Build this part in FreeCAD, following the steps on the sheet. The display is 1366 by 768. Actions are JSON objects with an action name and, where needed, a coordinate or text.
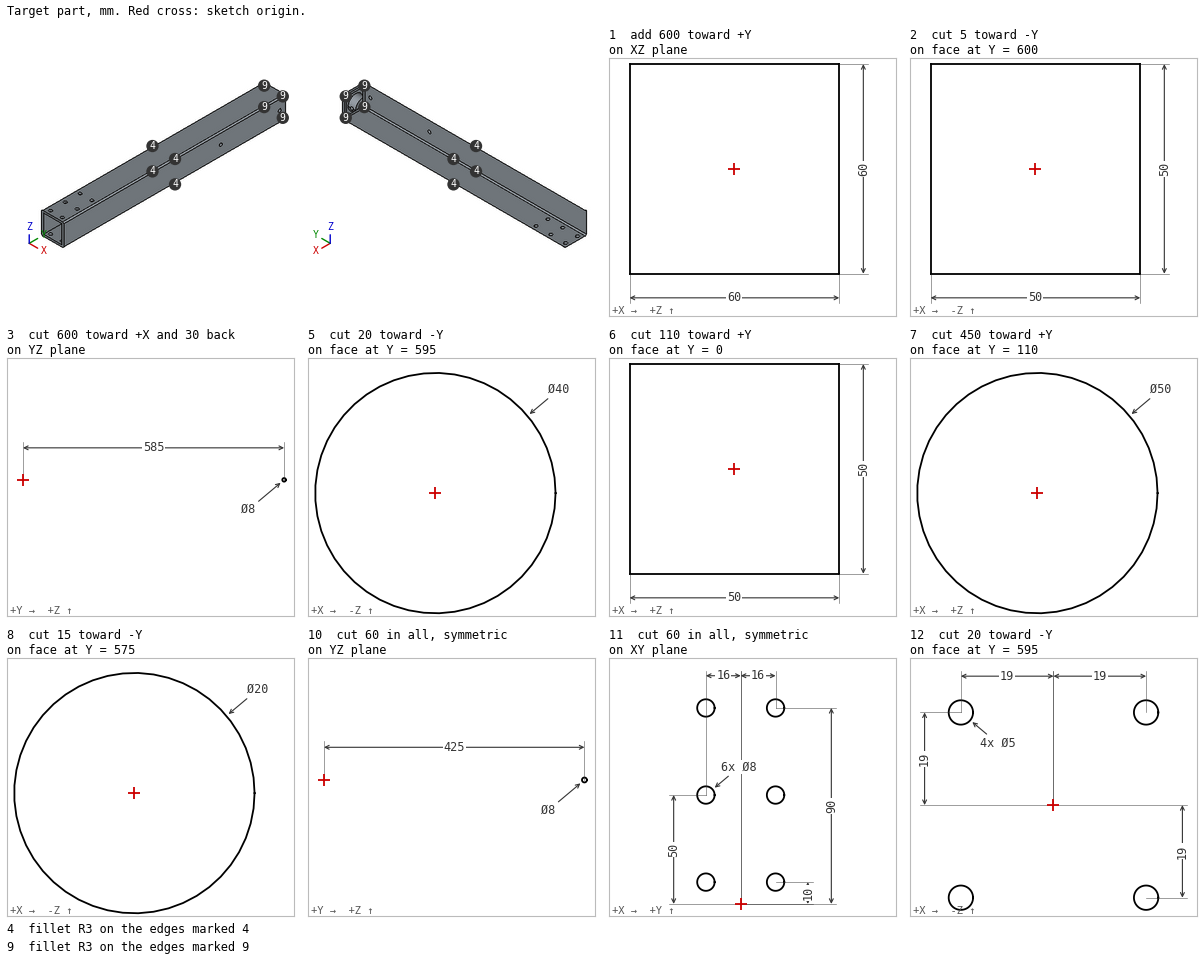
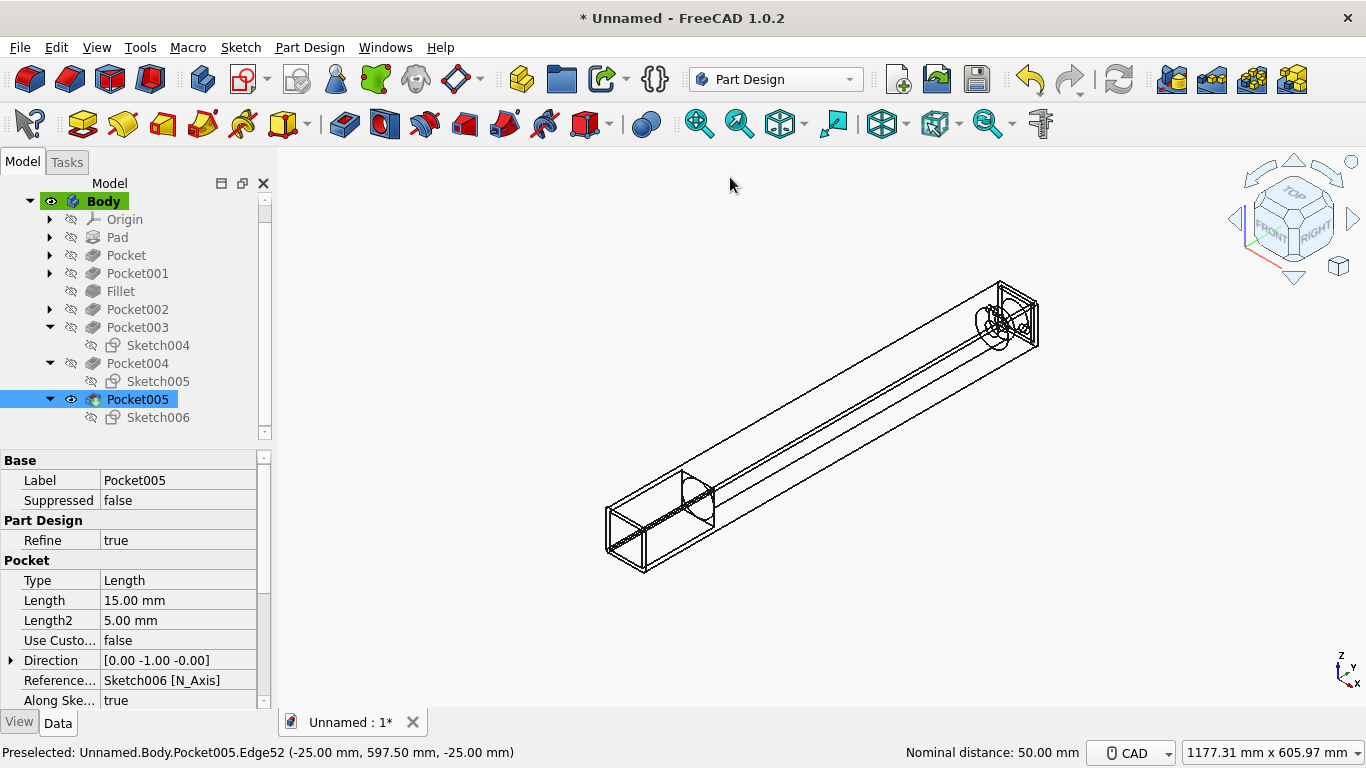
{"action": "key", "text": "2"}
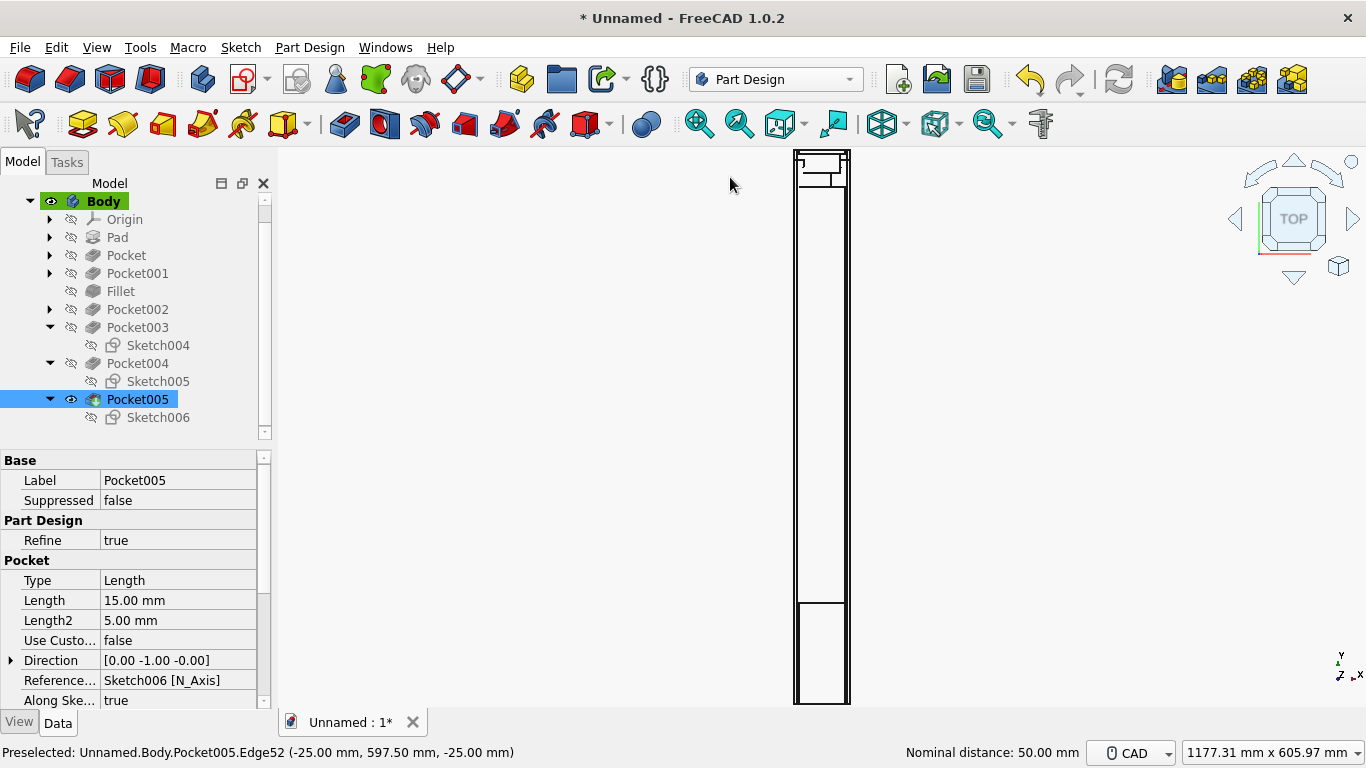
{"action": "key", "text": "1"}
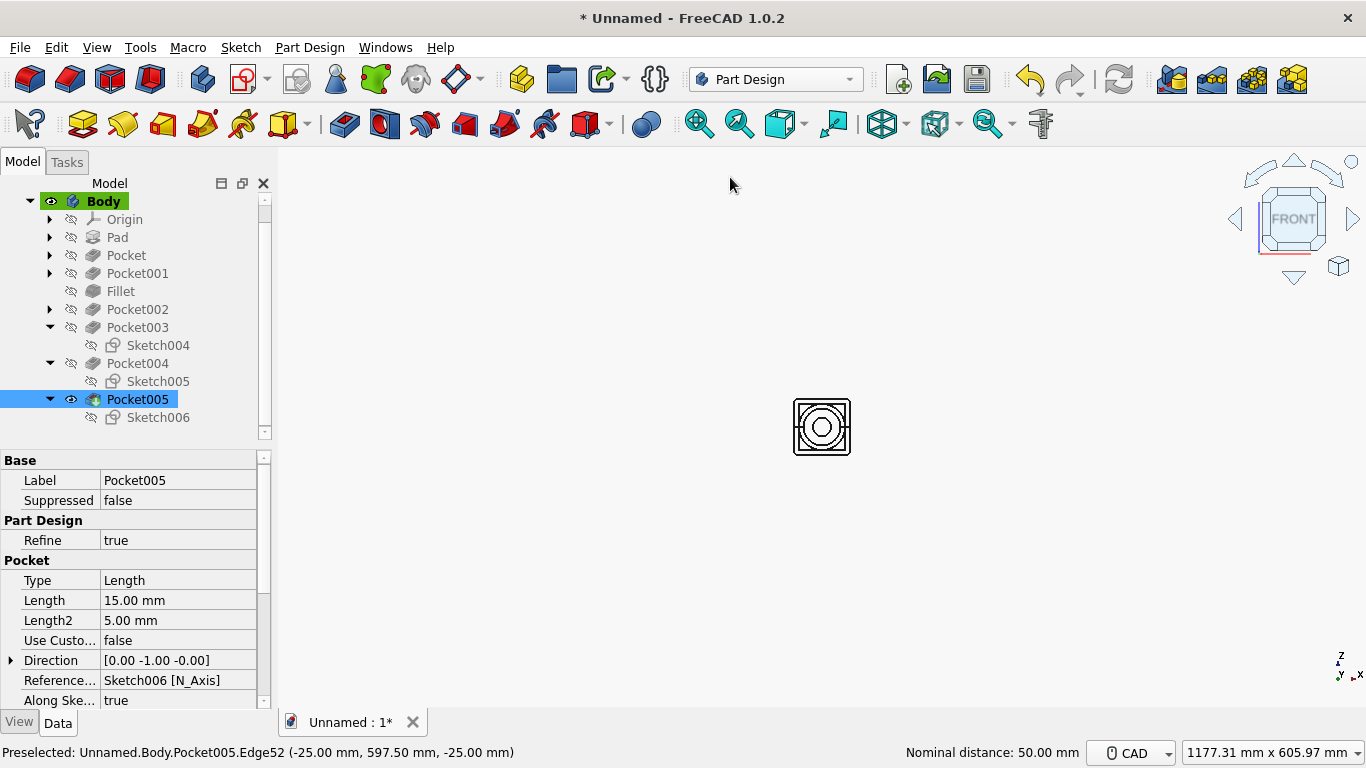
{"action": "left_click", "coordinate": [700, 124]}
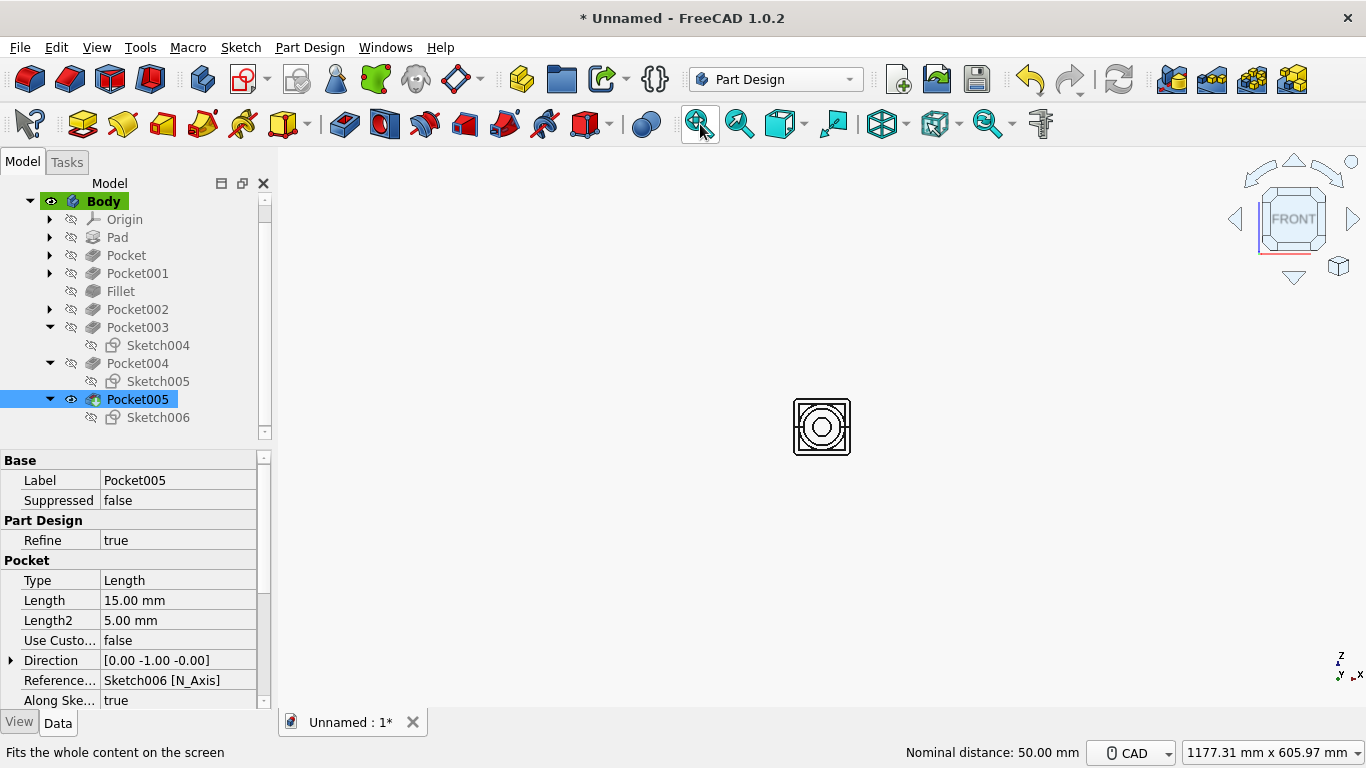
{"action": "scroll", "coordinate": [845, 403], "scroll_direction": "up", "scroll_amount": 11}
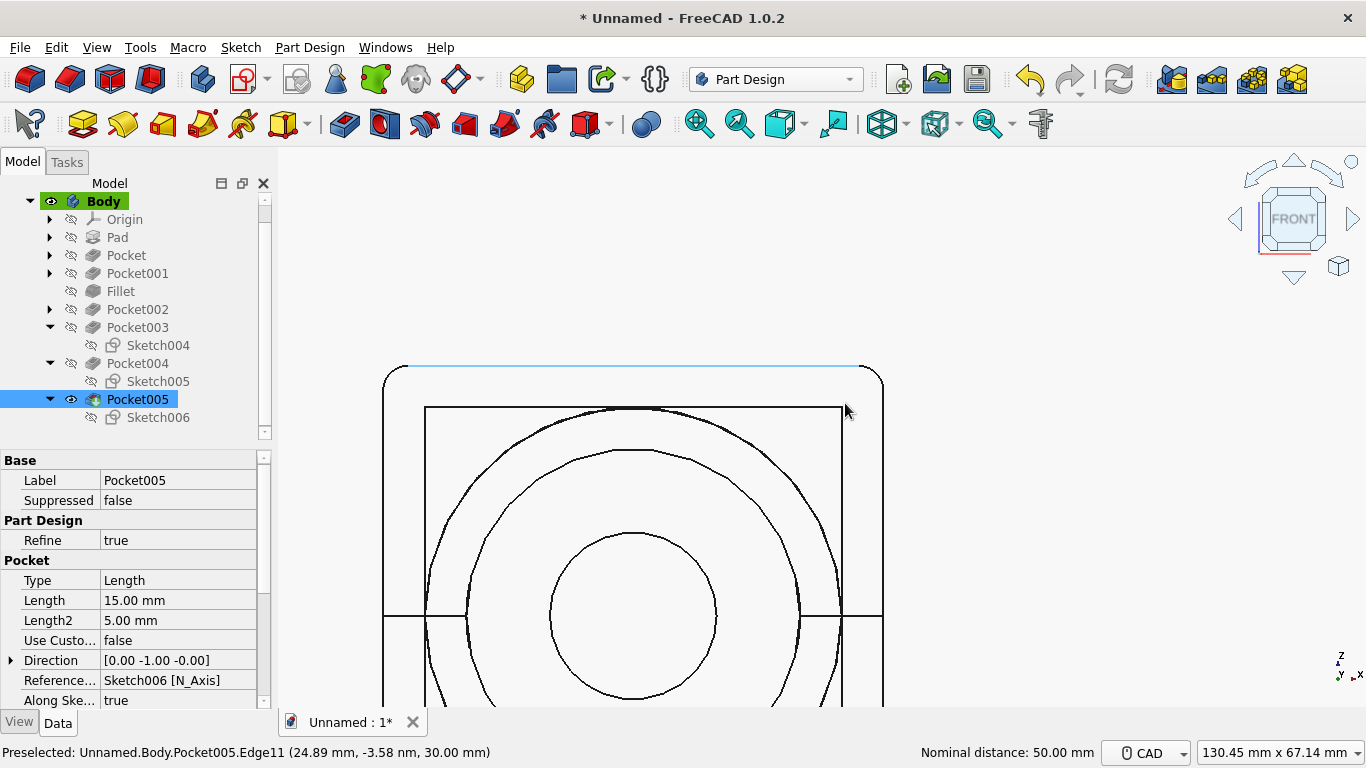
{"action": "left_click", "coordinate": [700, 124]}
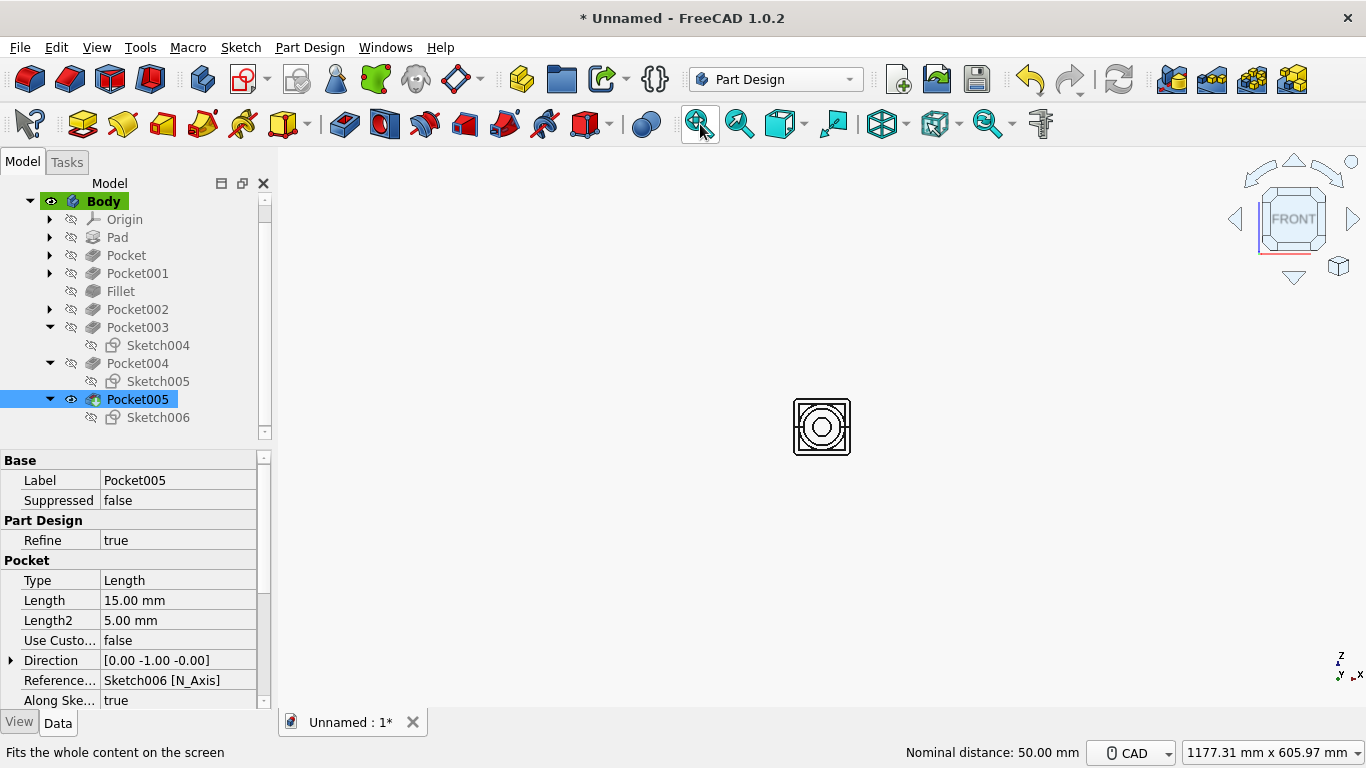
{"action": "key", "text": "3"}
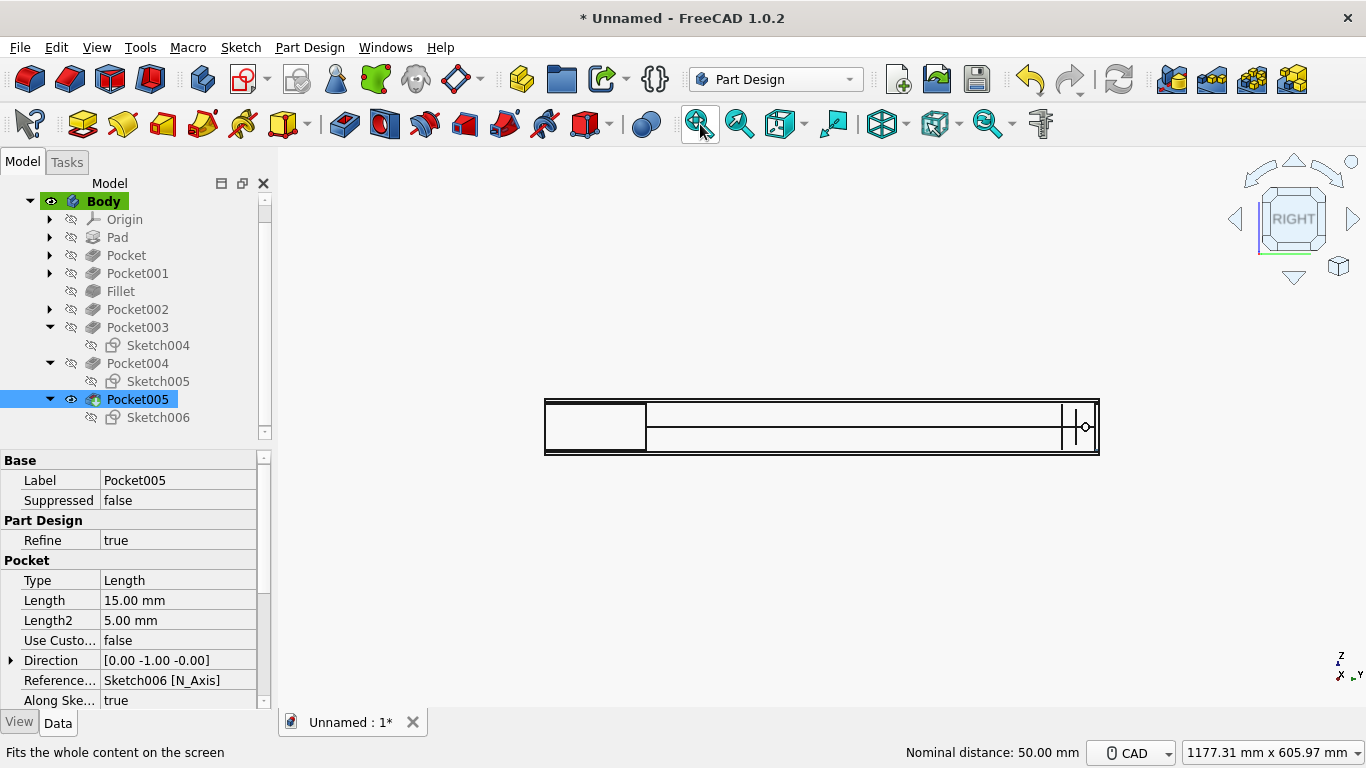
{"action": "scroll", "coordinate": [1097, 403], "scroll_direction": "up", "scroll_amount": 11}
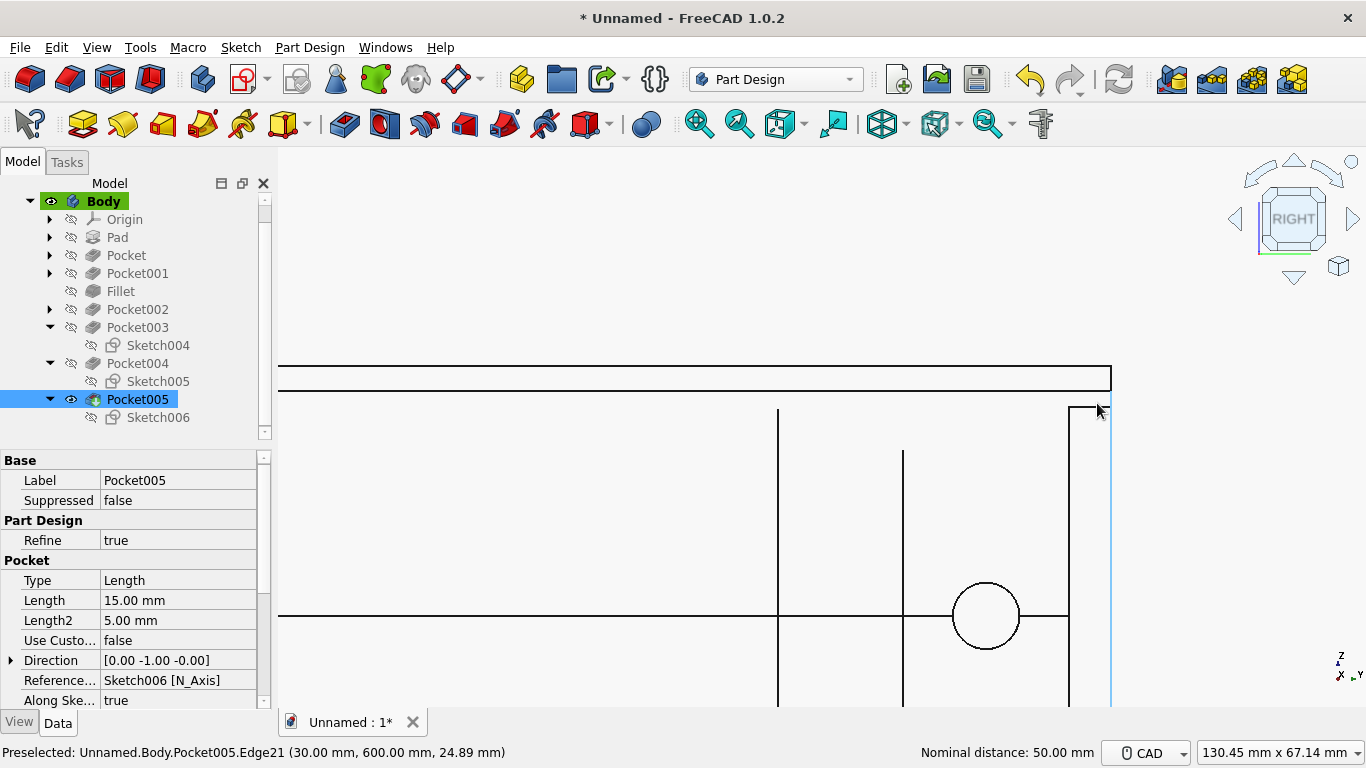
{"action": "left_click", "coordinate": [1090, 406], "text": "ctrl"}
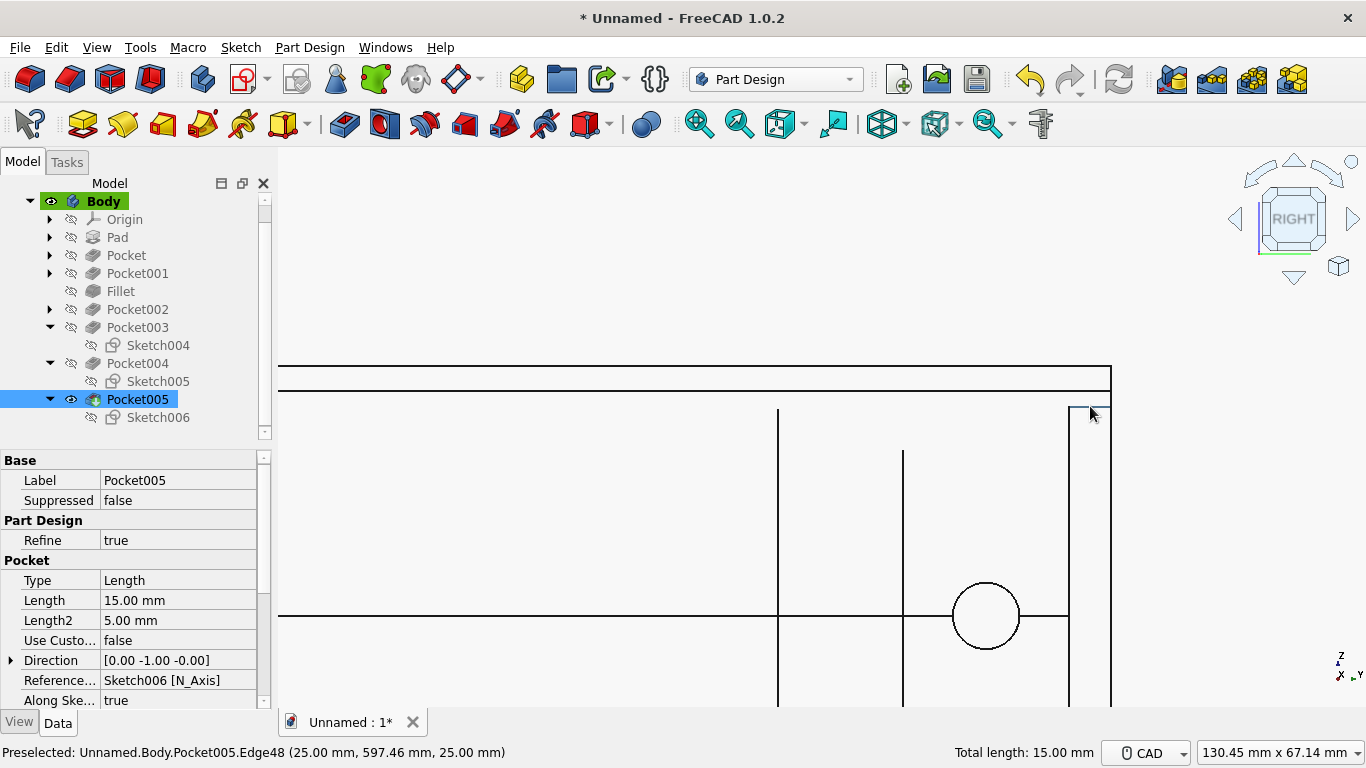
{"action": "left_click", "coordinate": [700, 124]}